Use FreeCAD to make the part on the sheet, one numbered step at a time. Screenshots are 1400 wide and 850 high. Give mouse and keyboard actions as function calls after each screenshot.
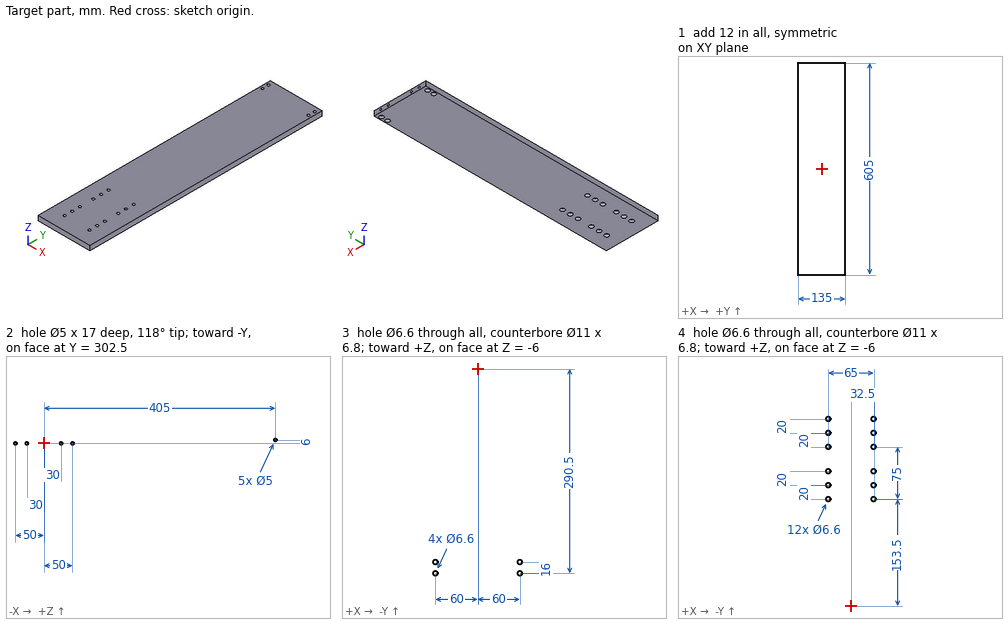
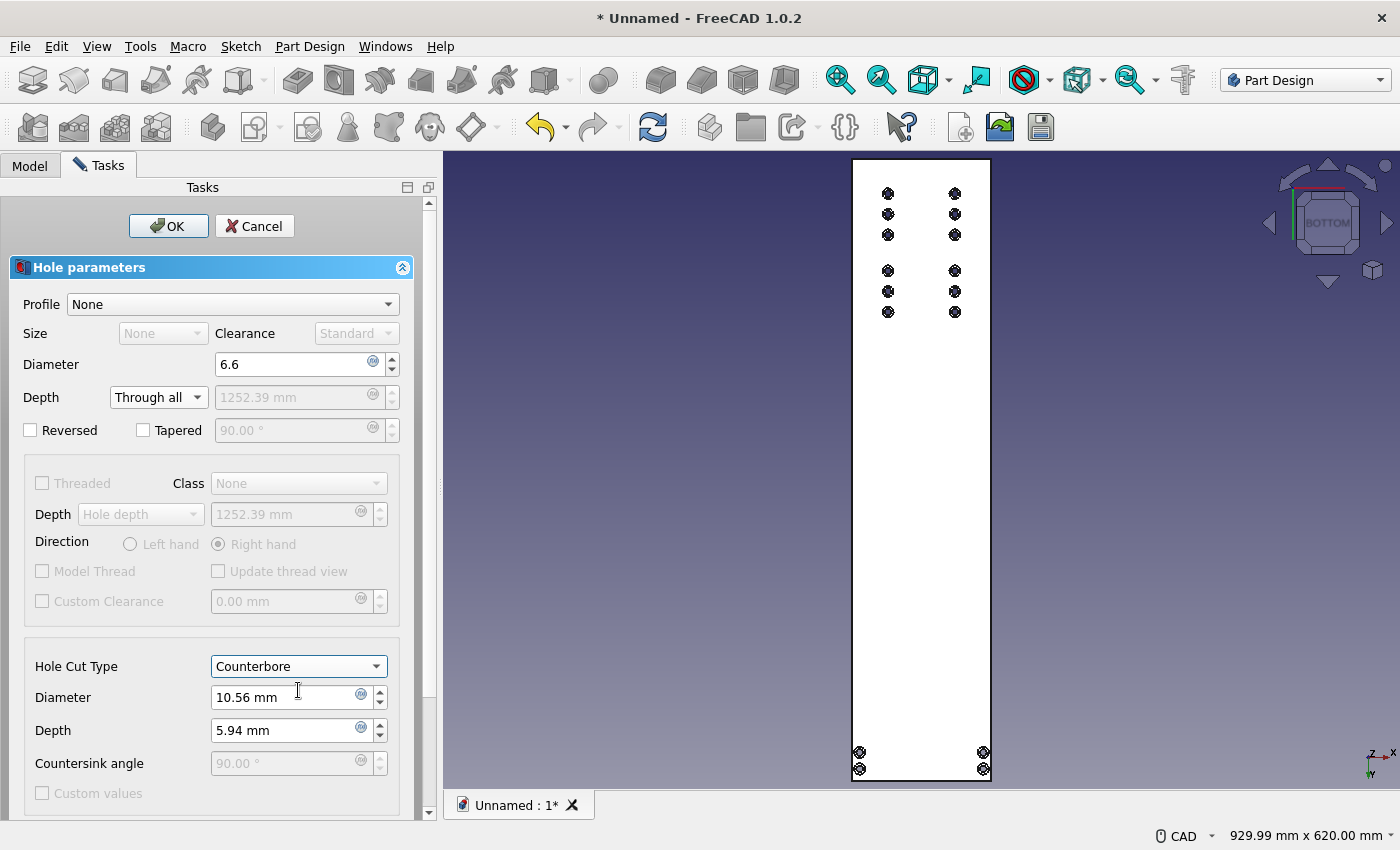
triple_click(292, 698)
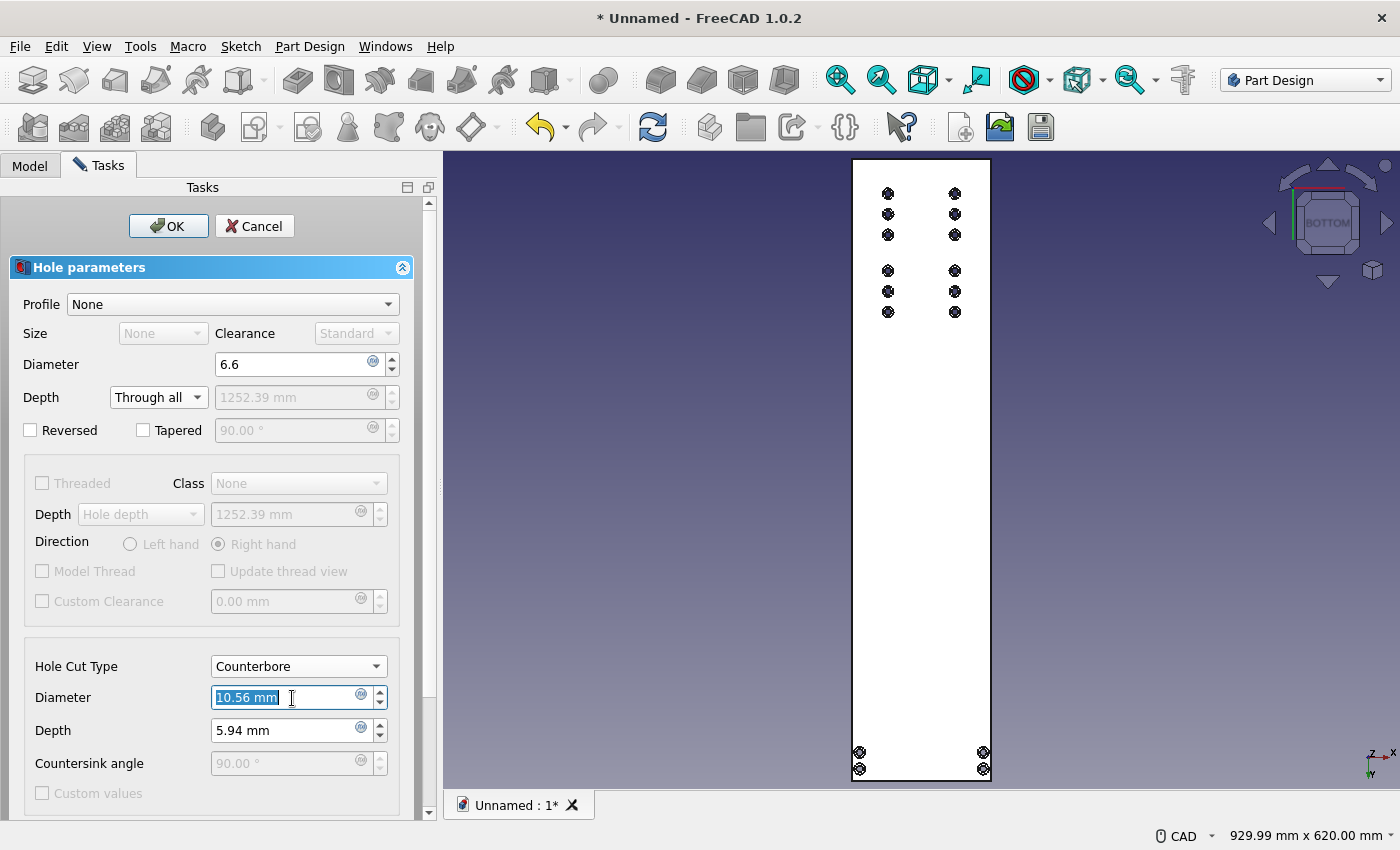
text(11)
key(Tab)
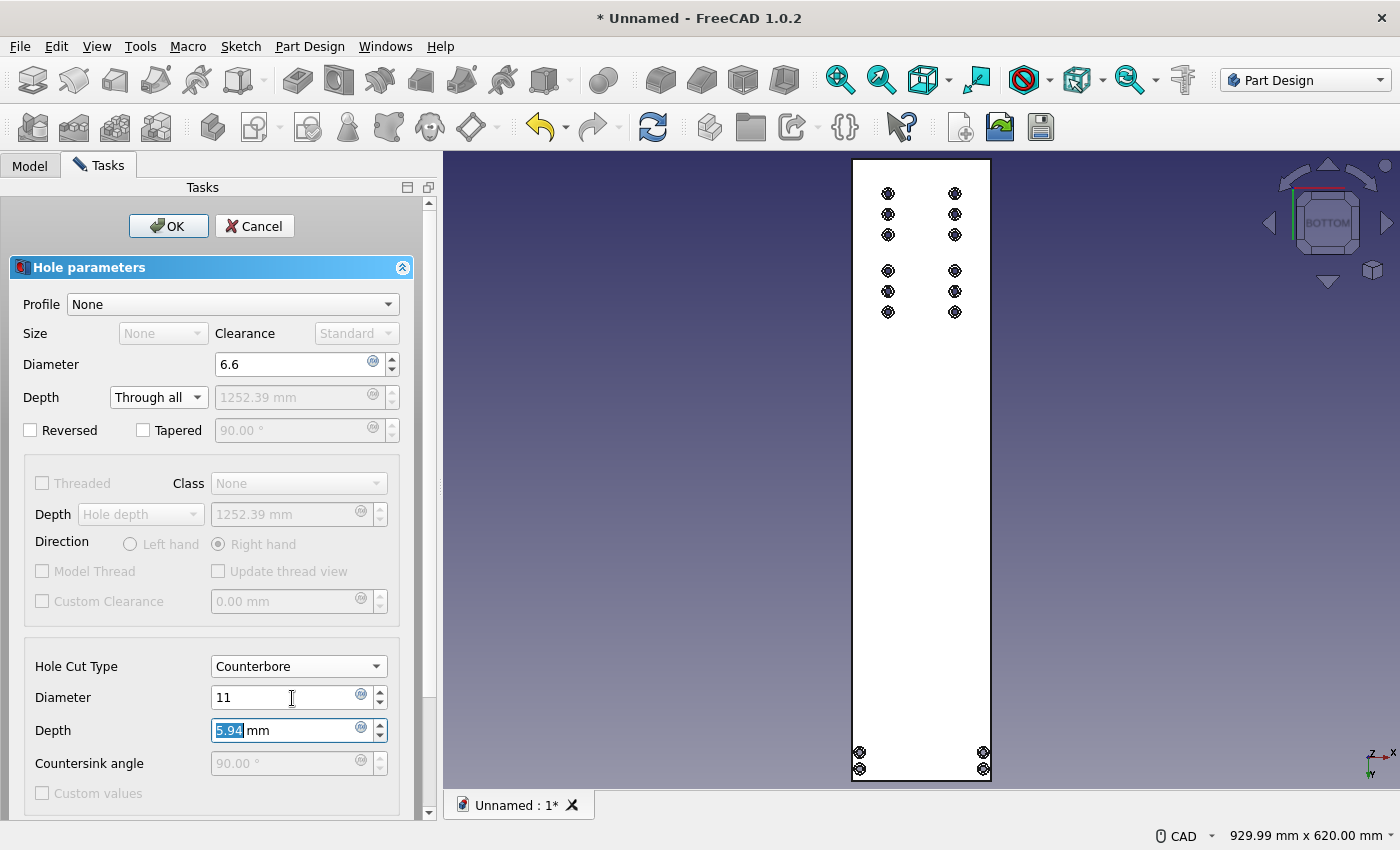
text(6.8)
key(Tab)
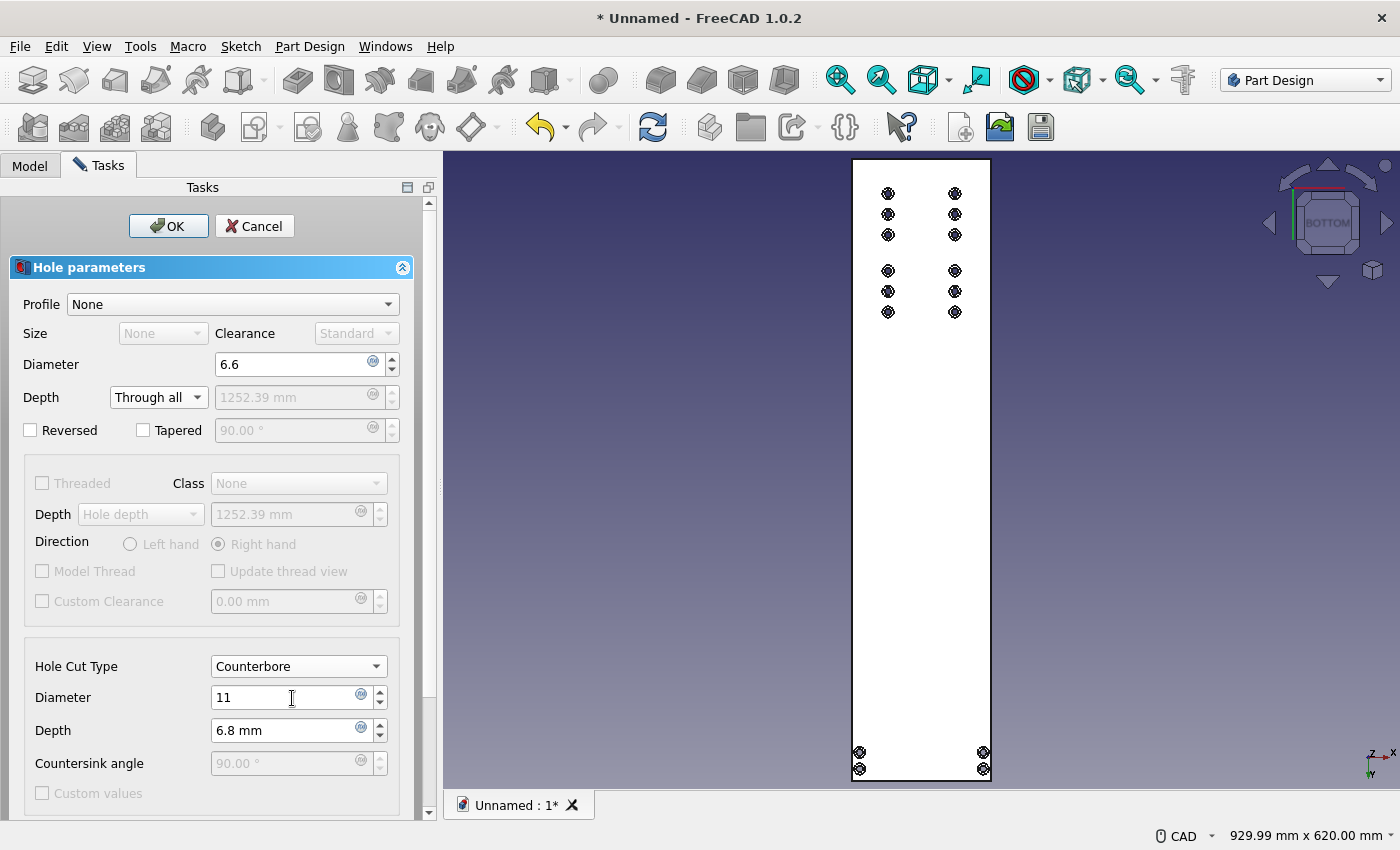
click(169, 226)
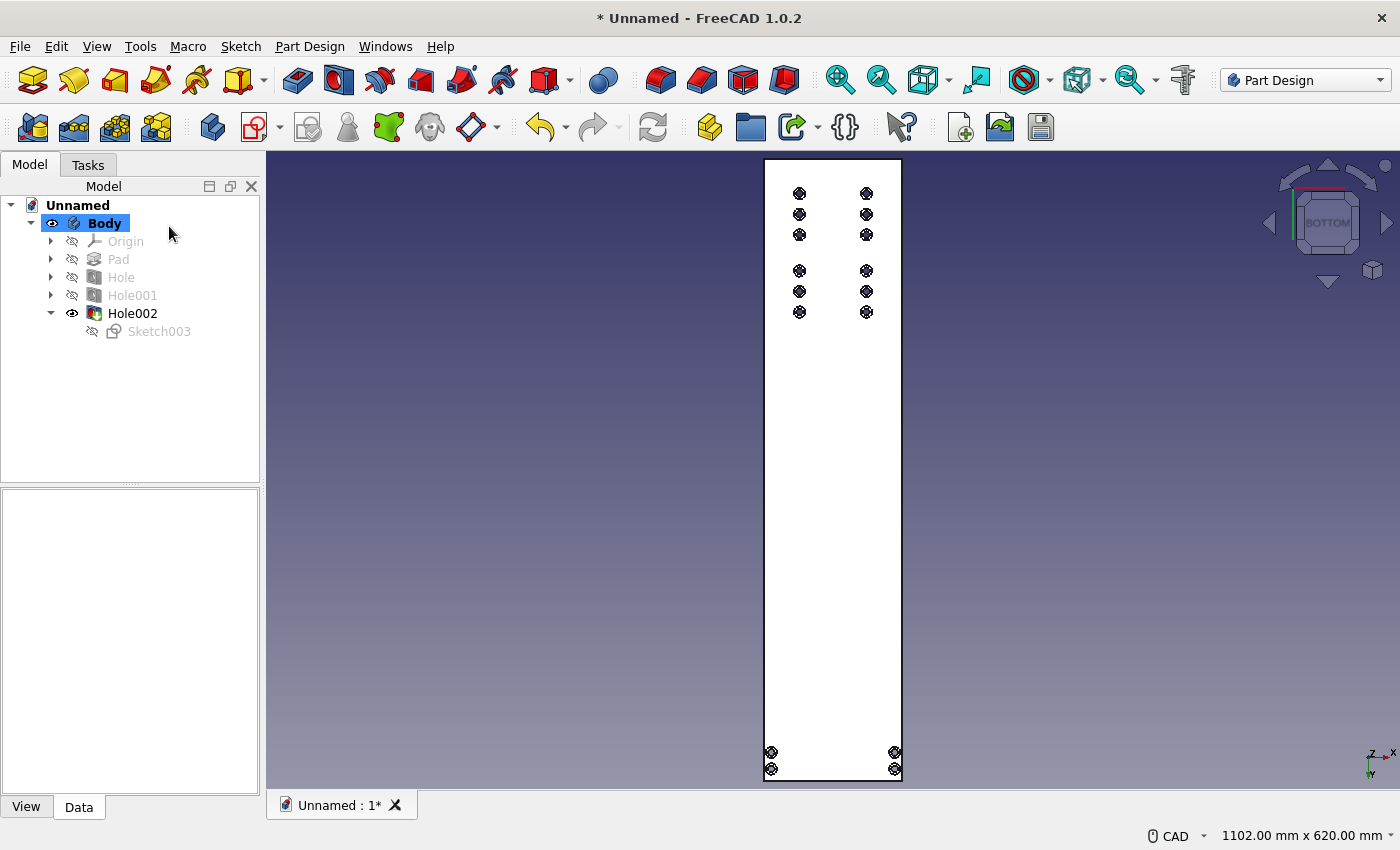
key(0)